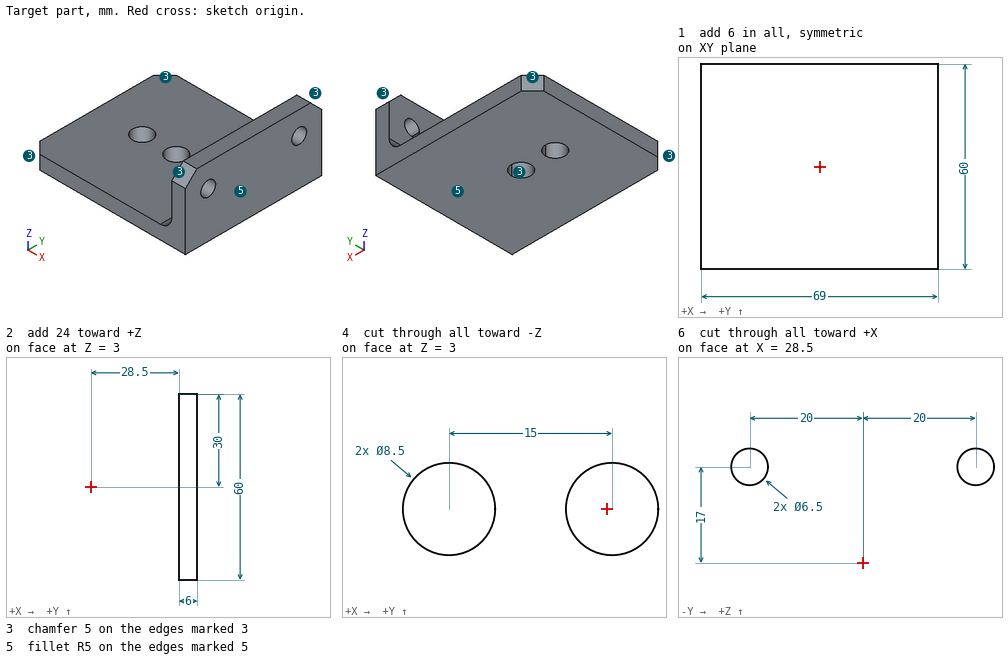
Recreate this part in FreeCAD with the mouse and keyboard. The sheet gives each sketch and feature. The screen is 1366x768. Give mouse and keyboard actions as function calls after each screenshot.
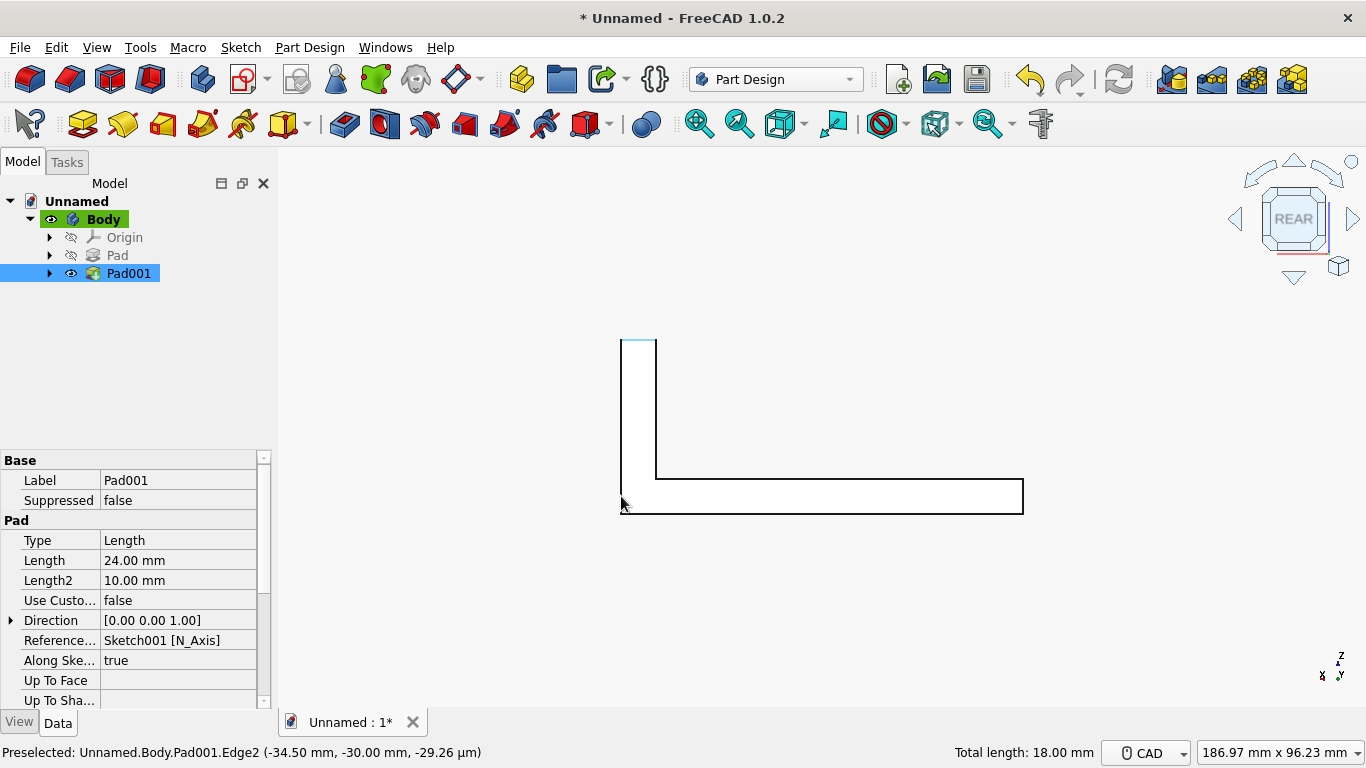
click(1023, 496, ctrl)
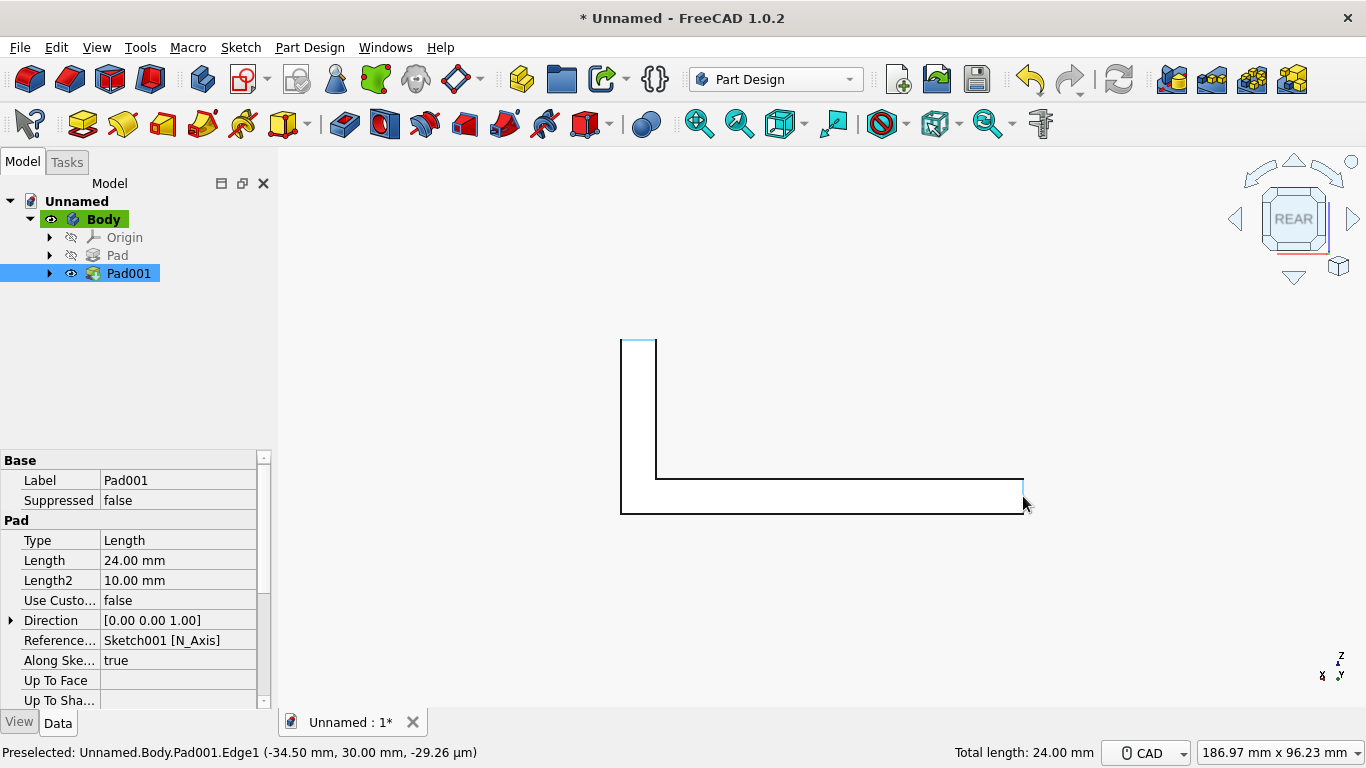
click(70, 80)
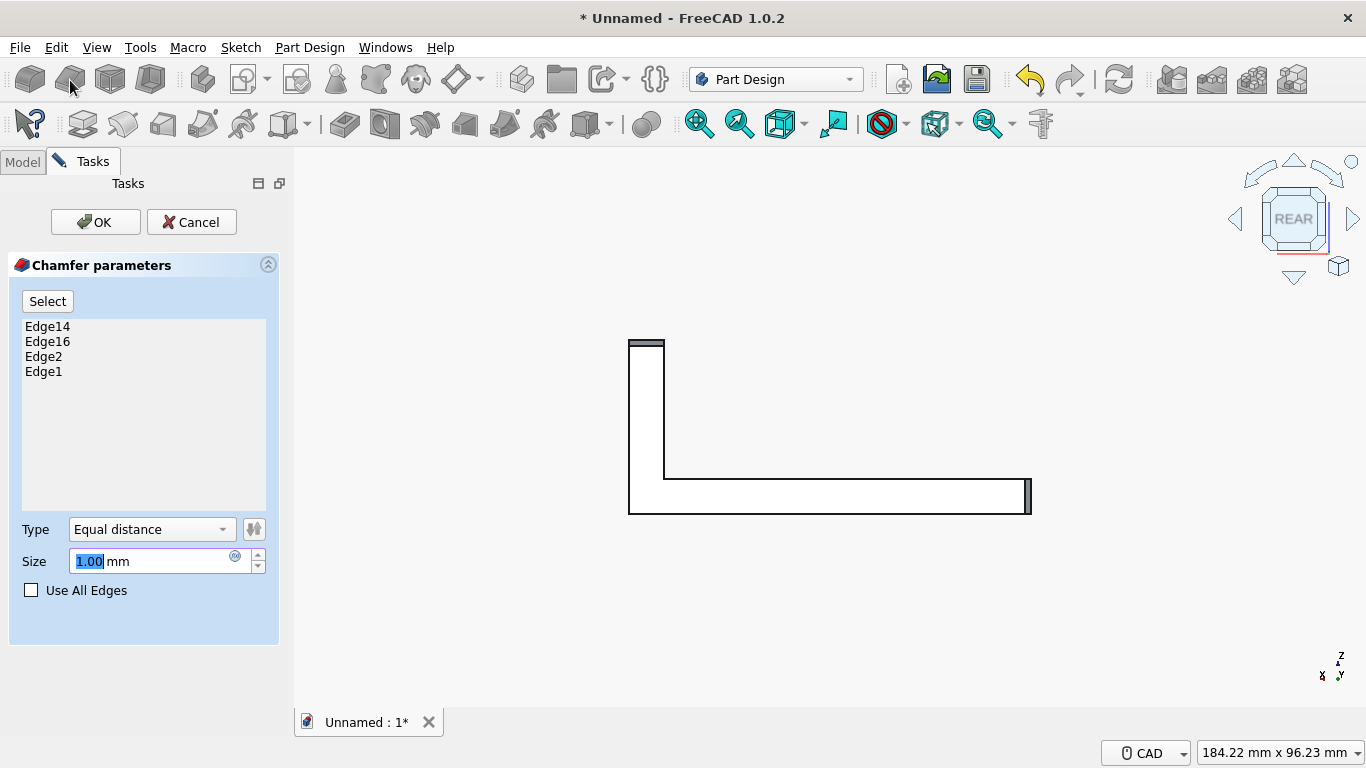
text(5)
key(Tab)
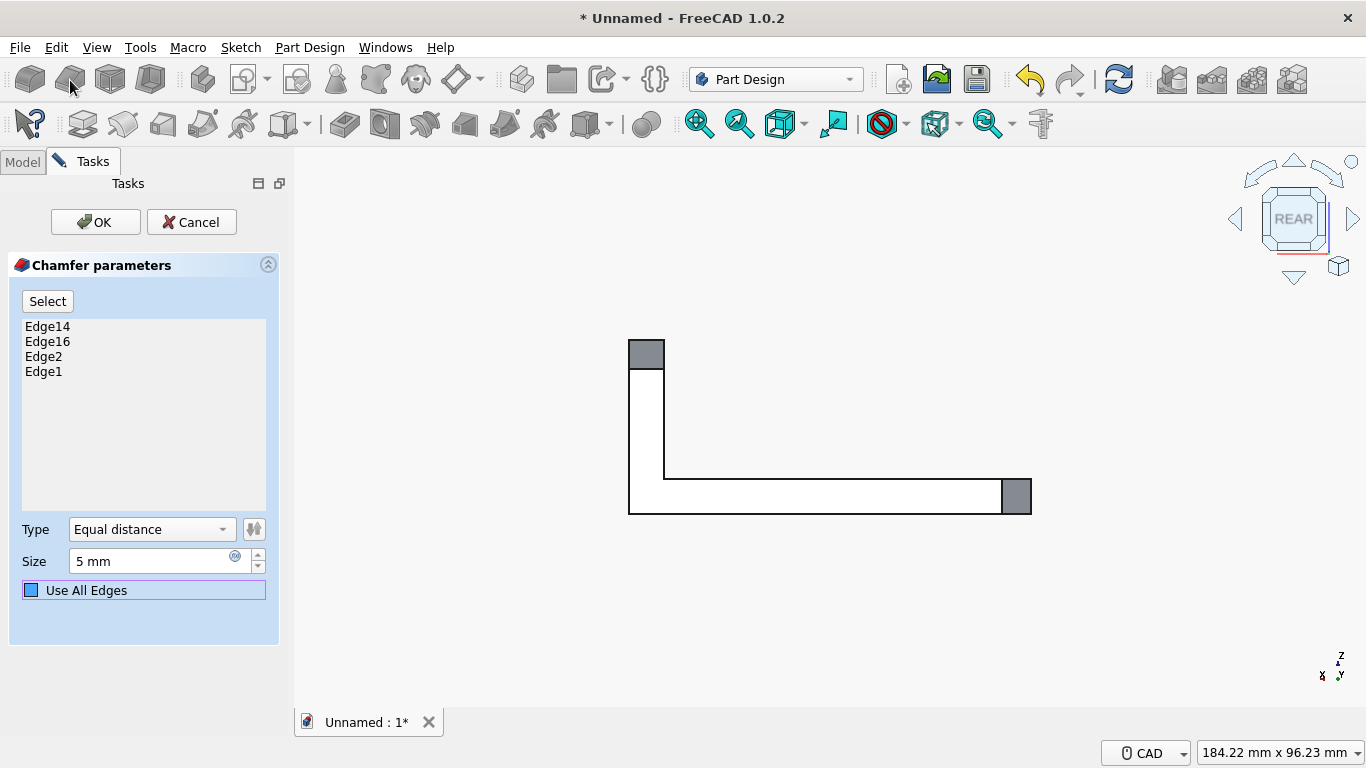
click(96, 222)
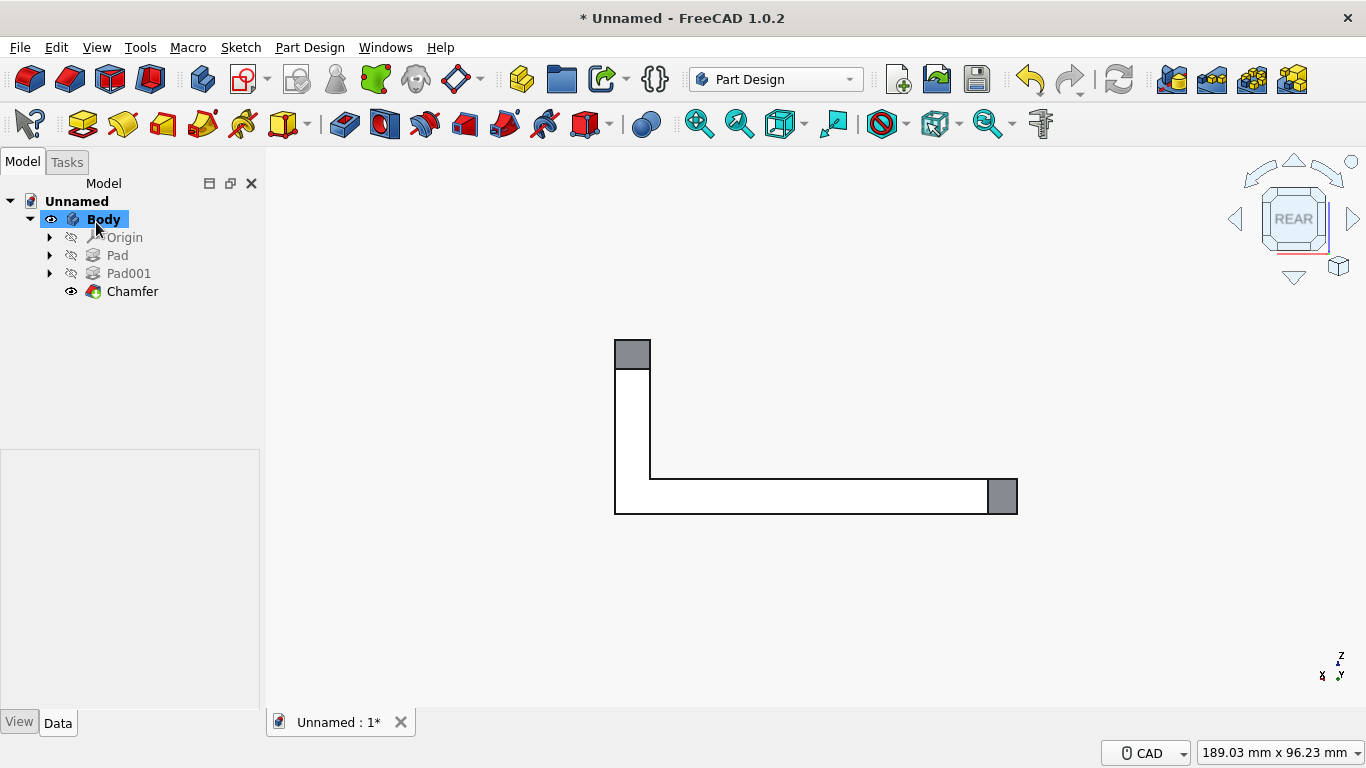
click(700, 124)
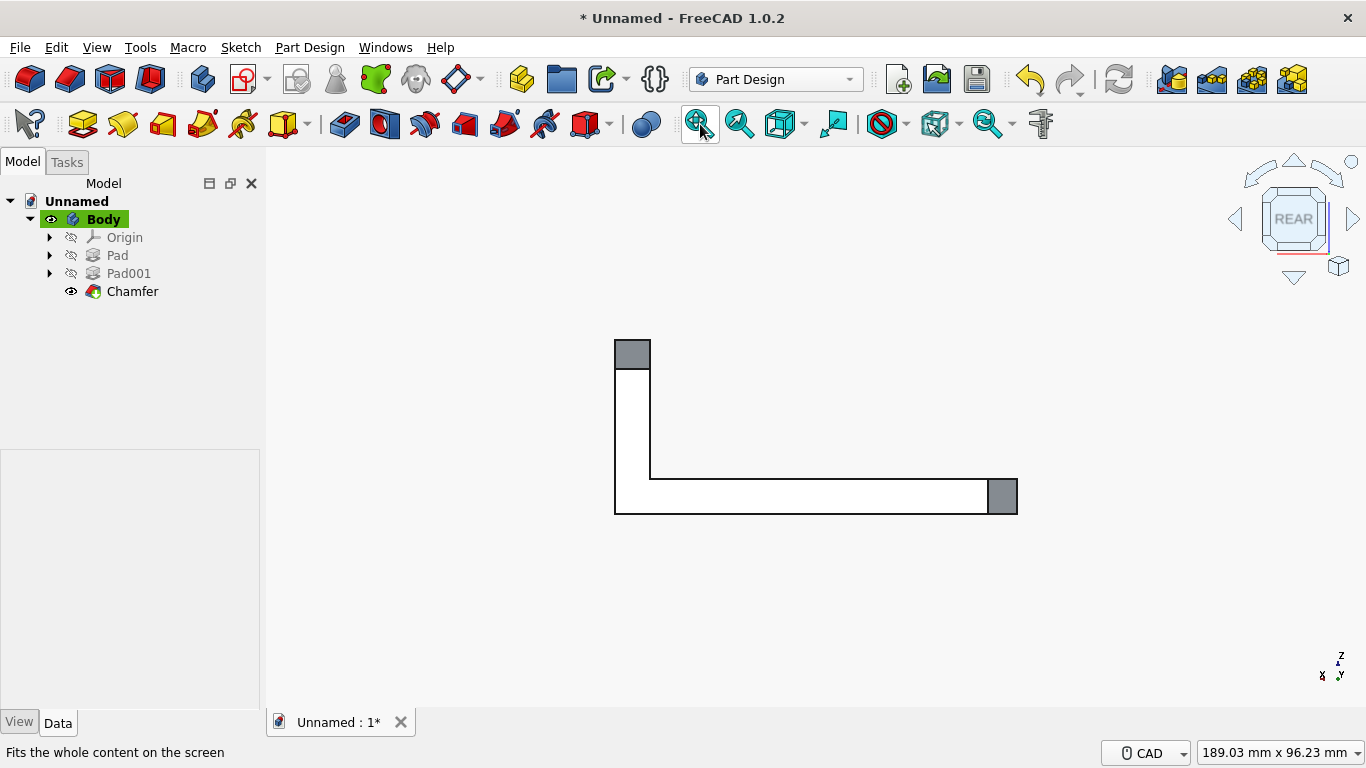
key(0)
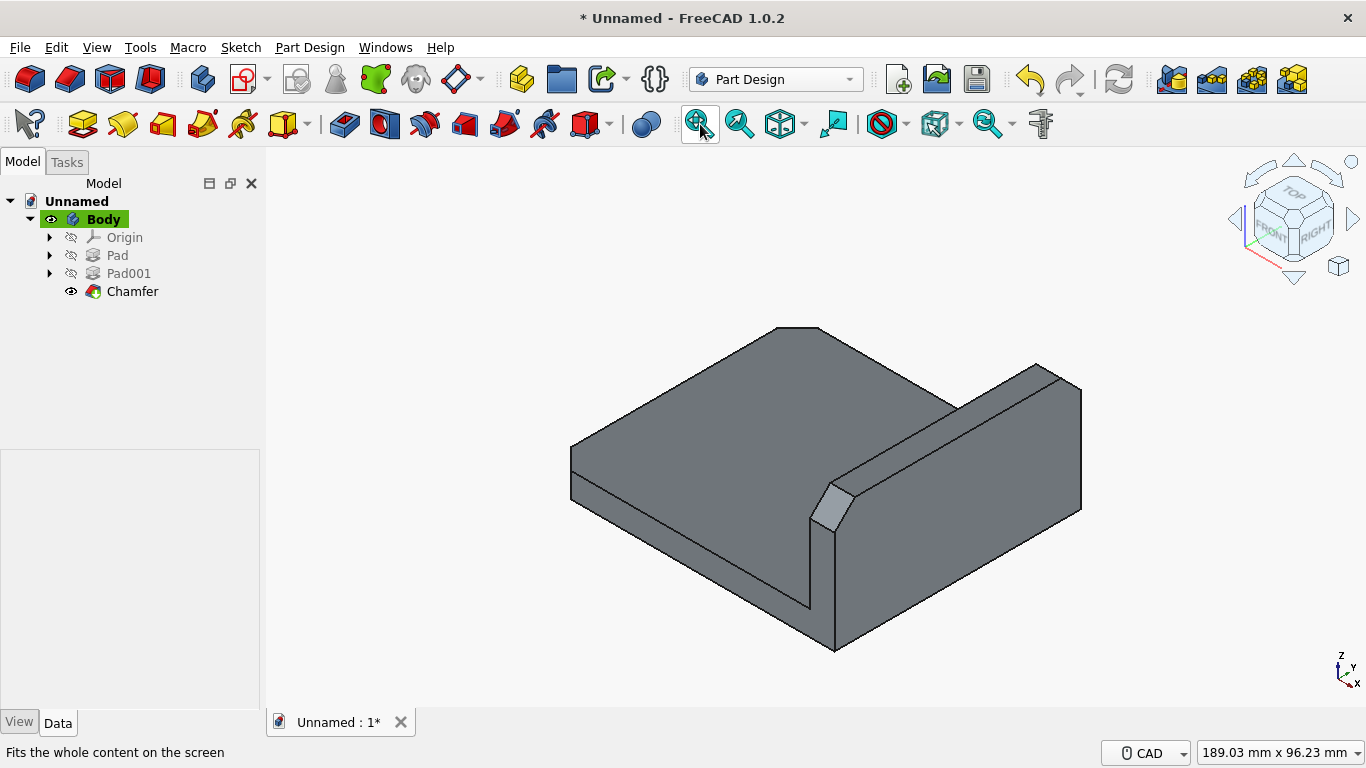
click(804, 462)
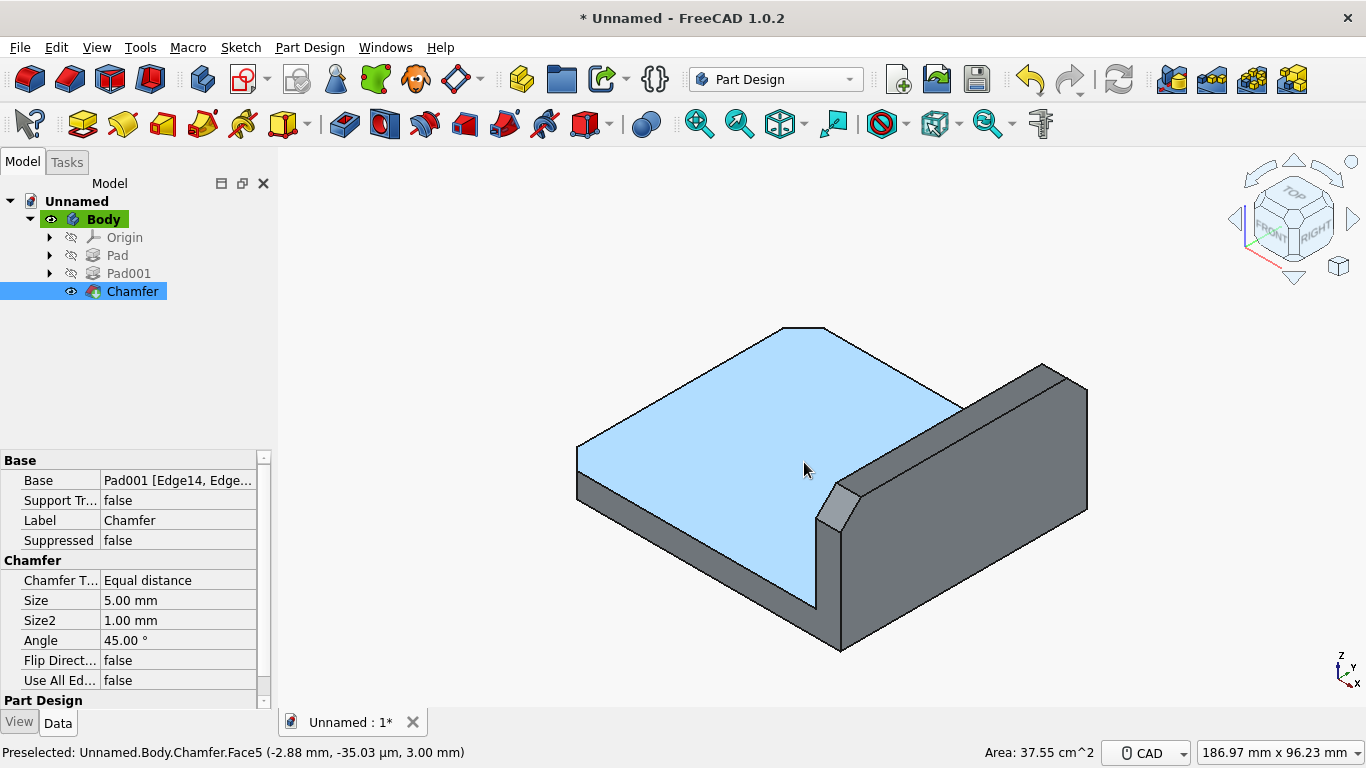
click(244, 80)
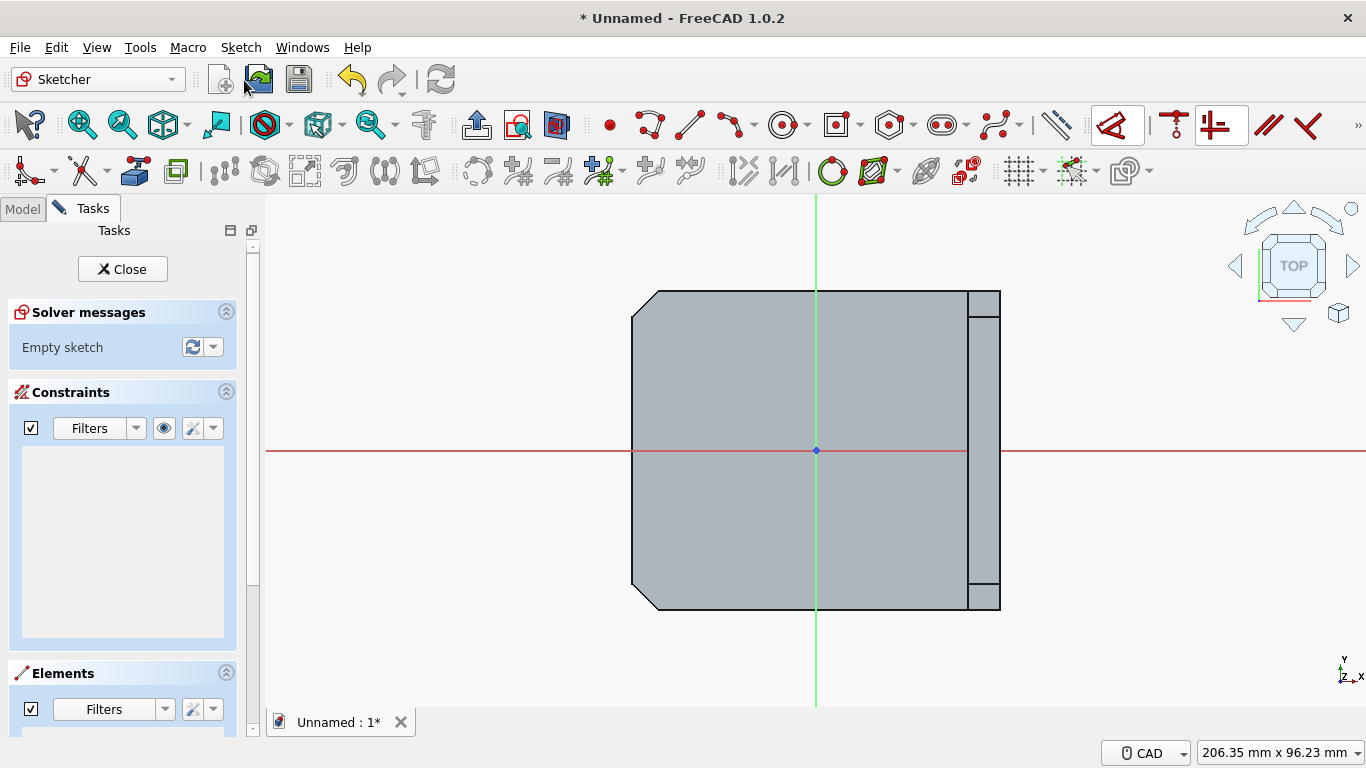
scroll(787, 451, up, 8)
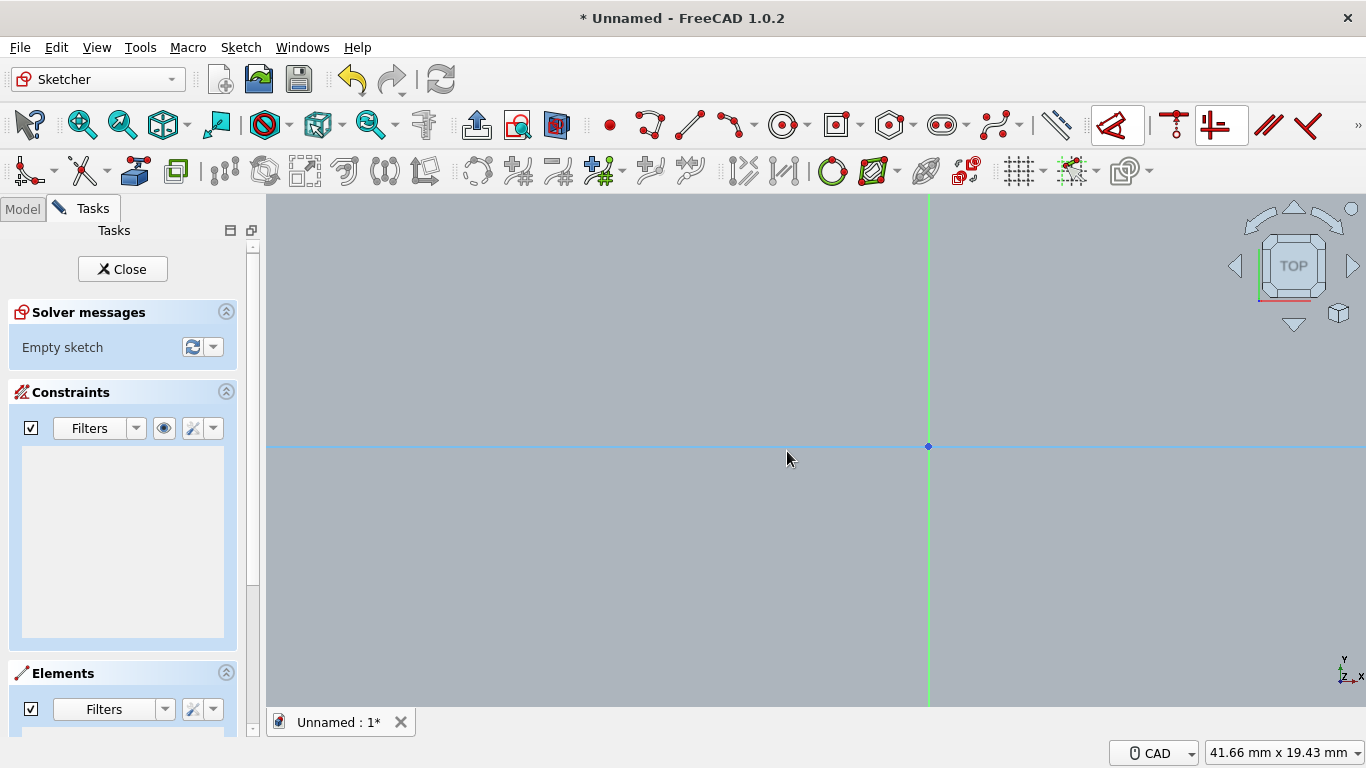
click(784, 126)